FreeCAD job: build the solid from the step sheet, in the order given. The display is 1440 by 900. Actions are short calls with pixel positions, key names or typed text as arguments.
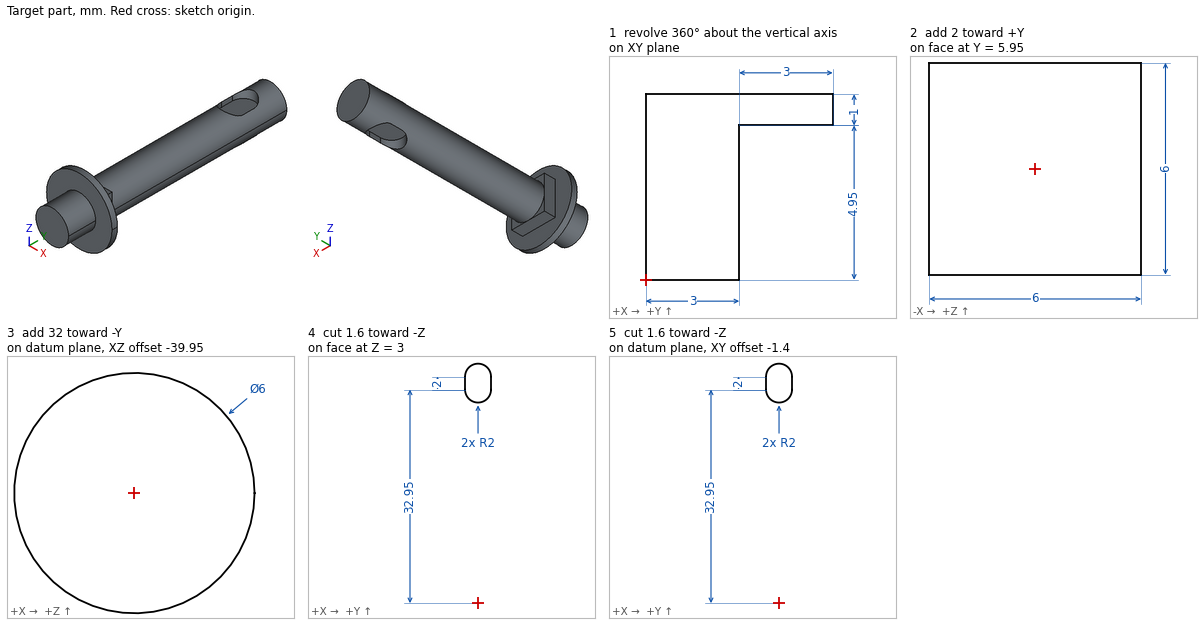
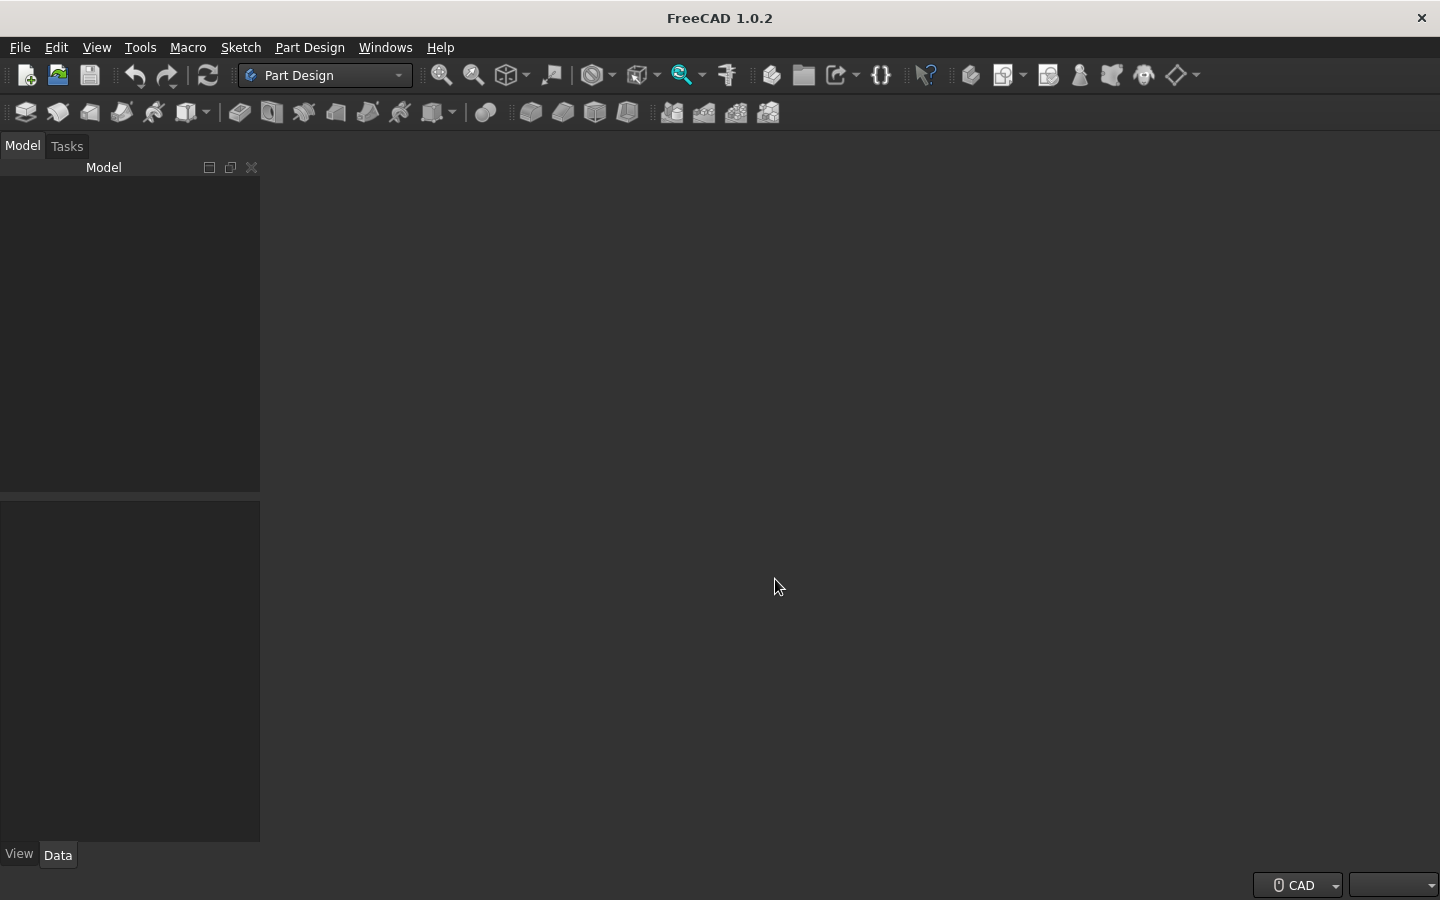
click(26, 76)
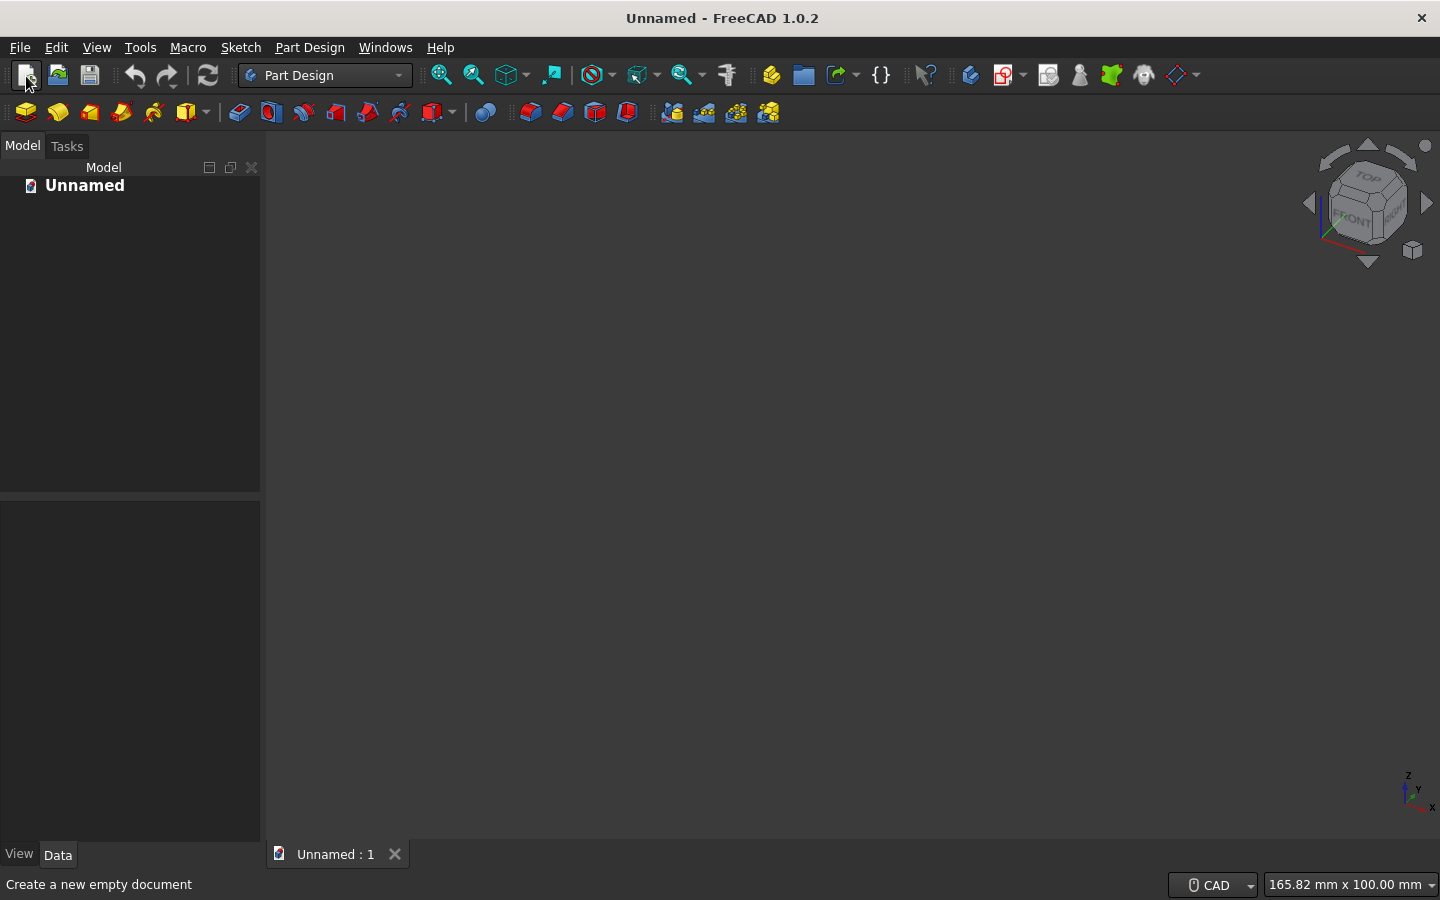
click(1004, 76)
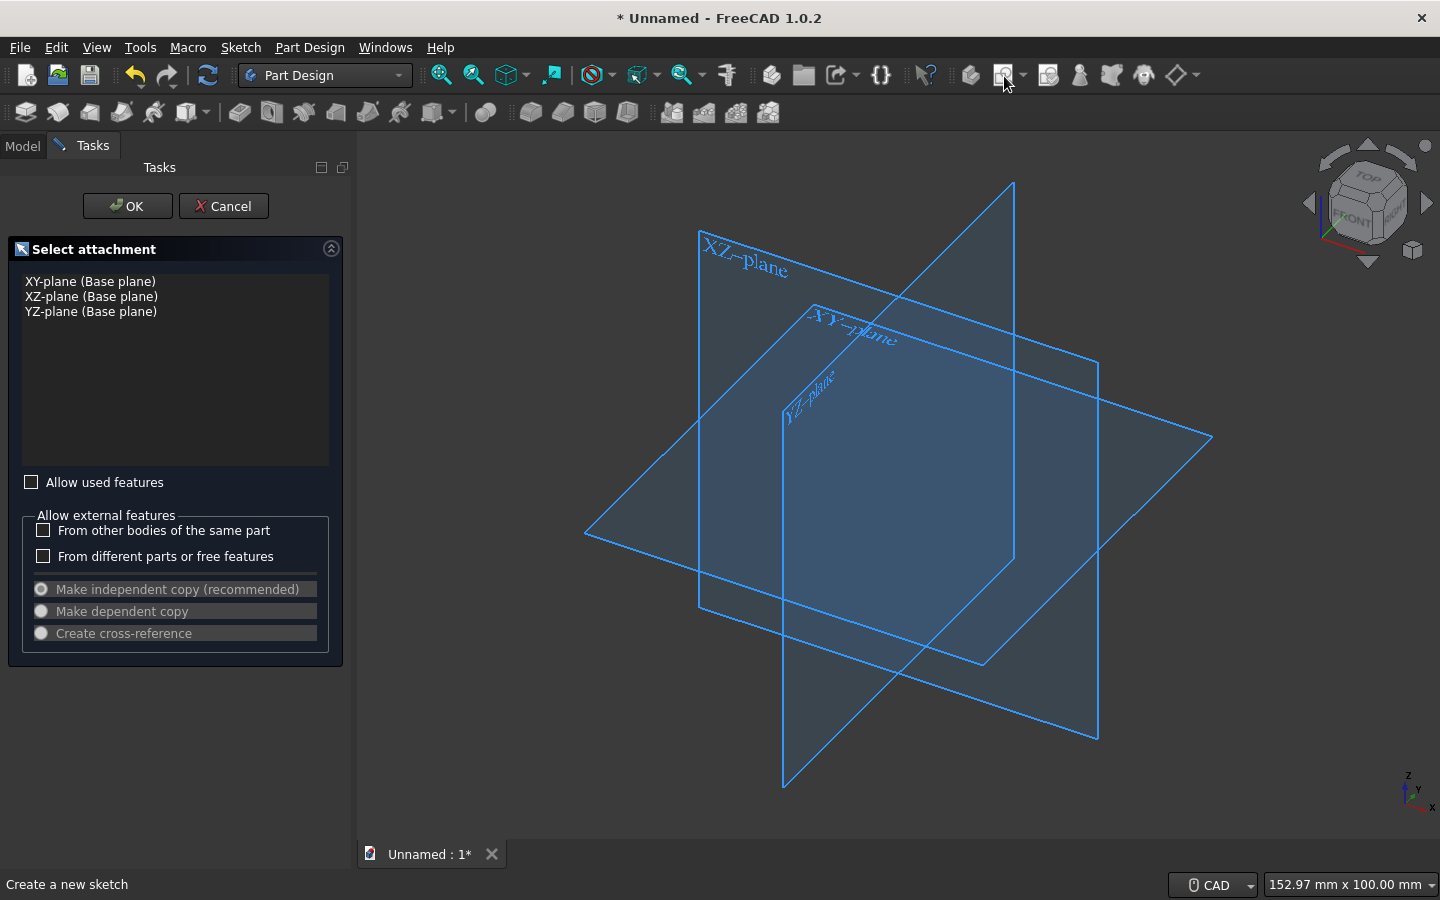
click(82, 282)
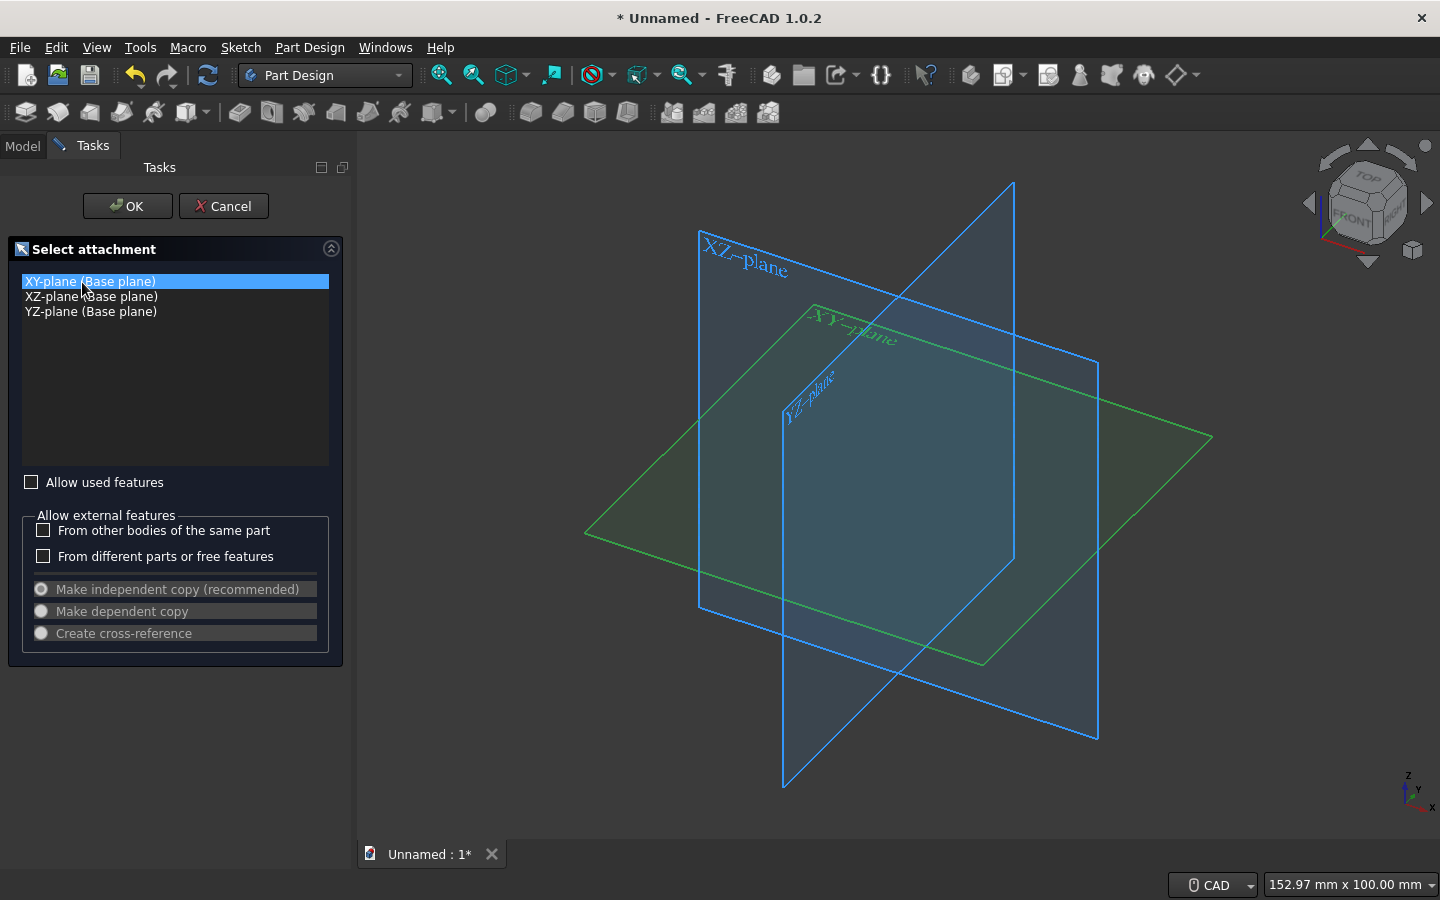
click(128, 206)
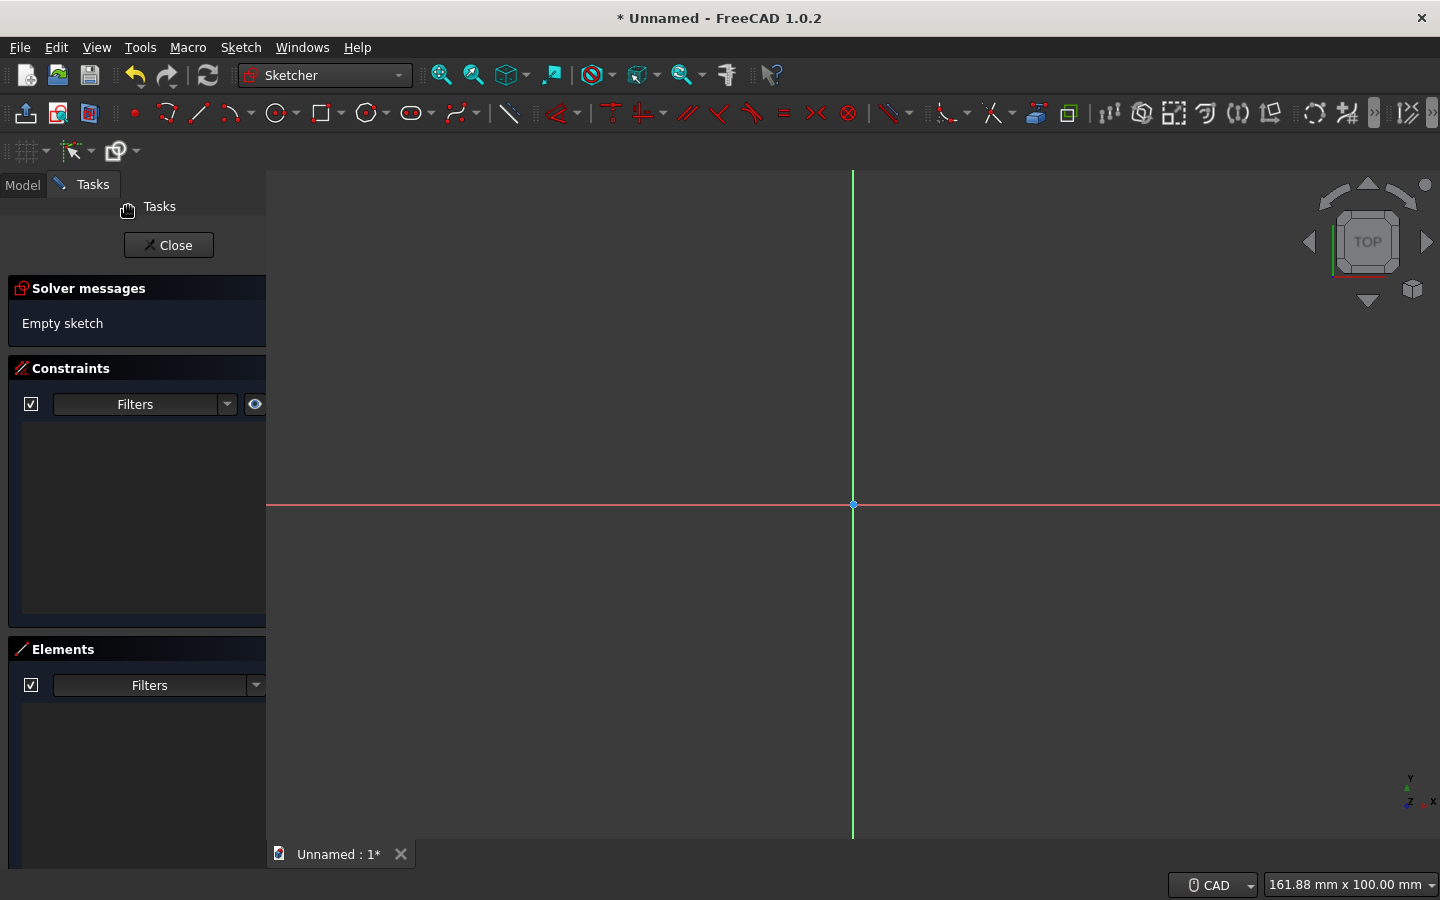
scroll(882, 483, up, 12)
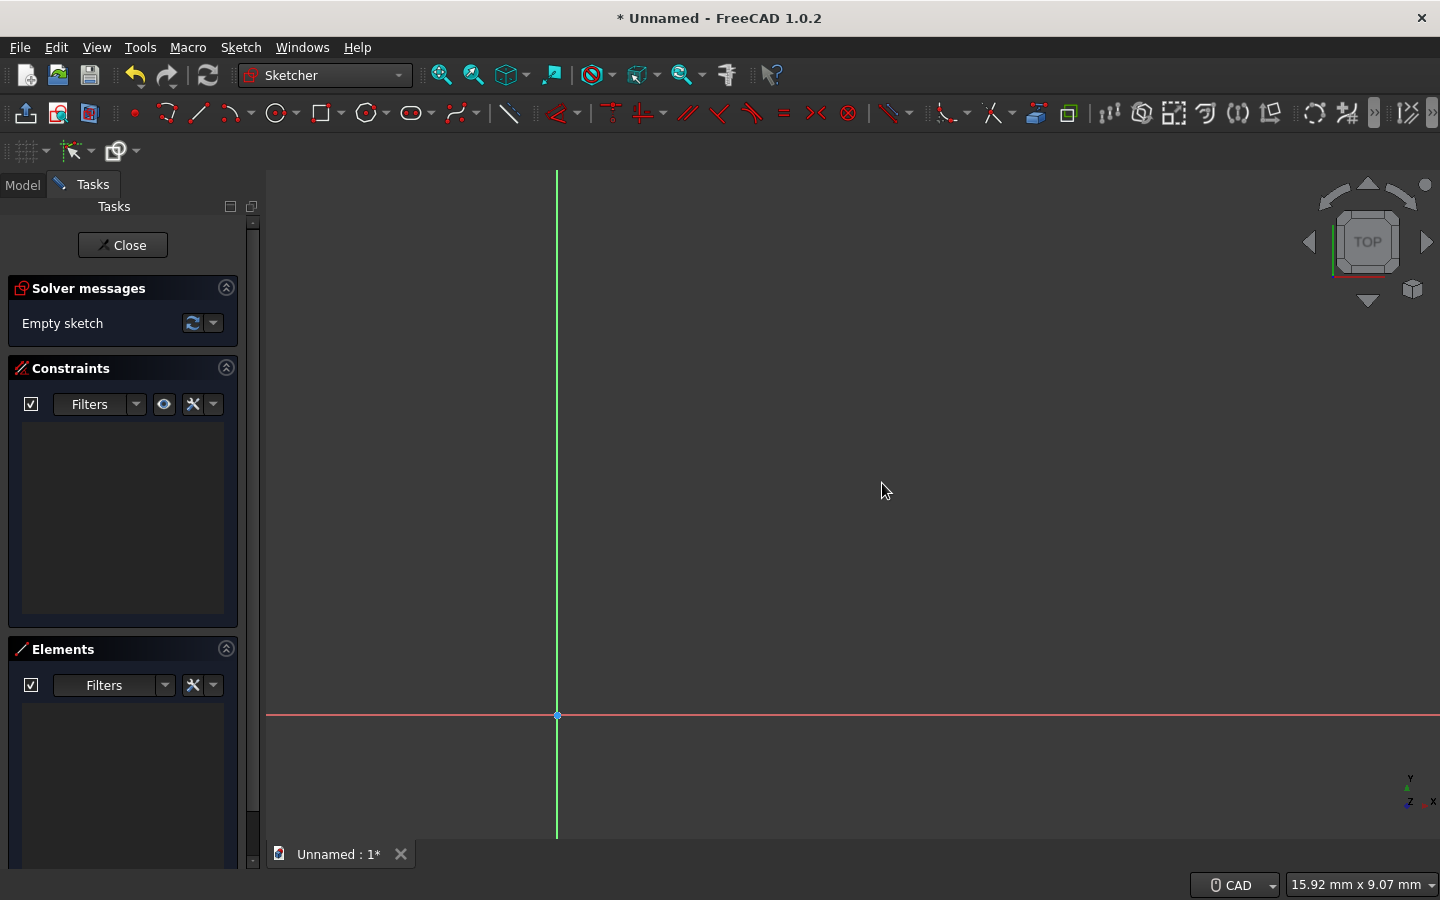
click(168, 114)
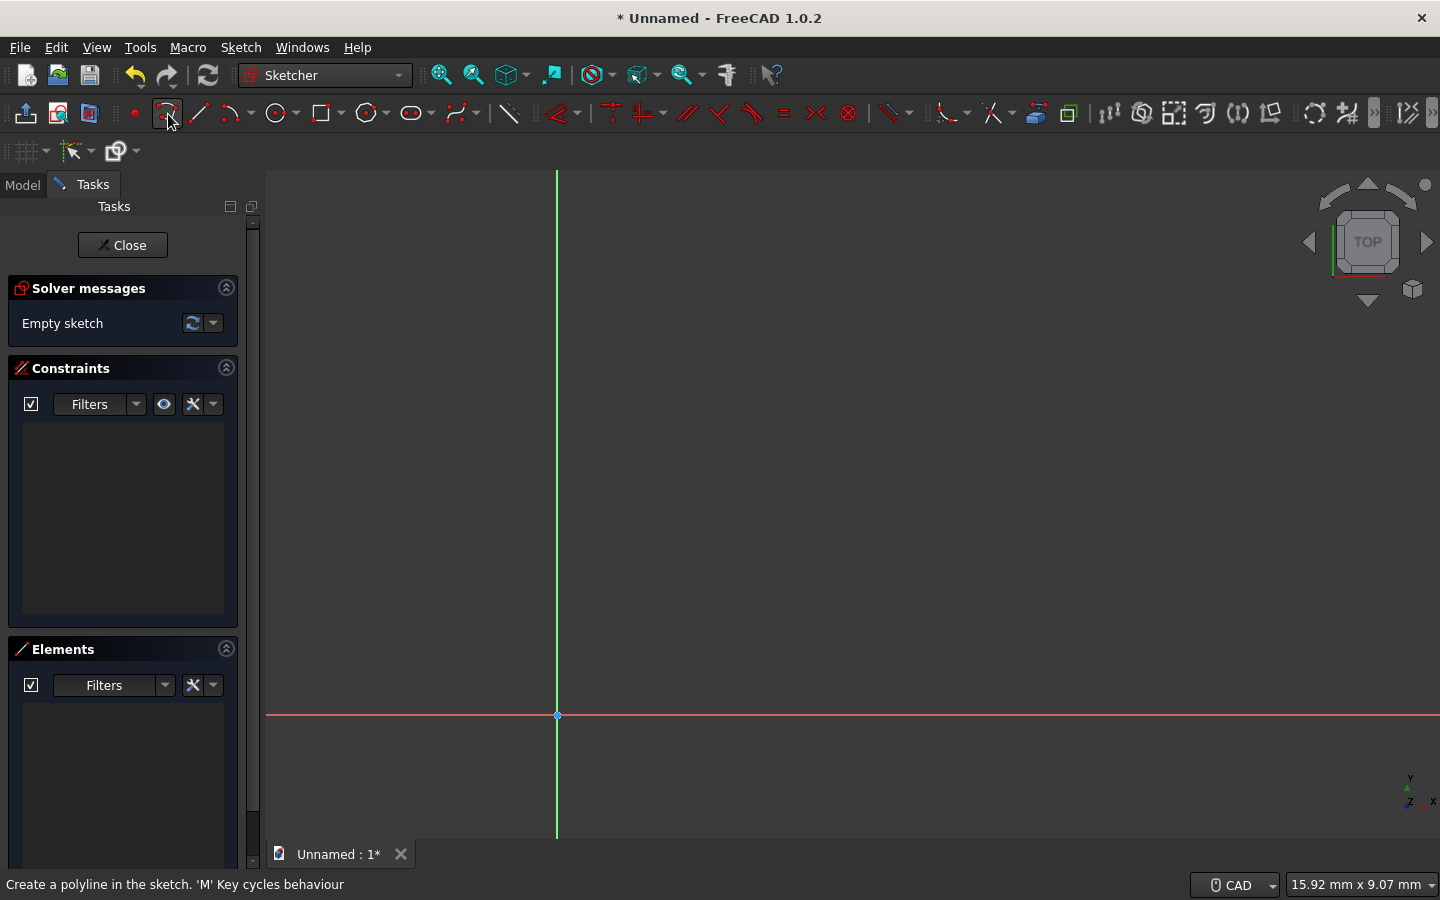
click(557, 715)
click(778, 706)
click(778, 350)
click(1000, 350)
click(1000, 277)
click(566, 277)
click(557, 715)
key(Escape)
key(Escape)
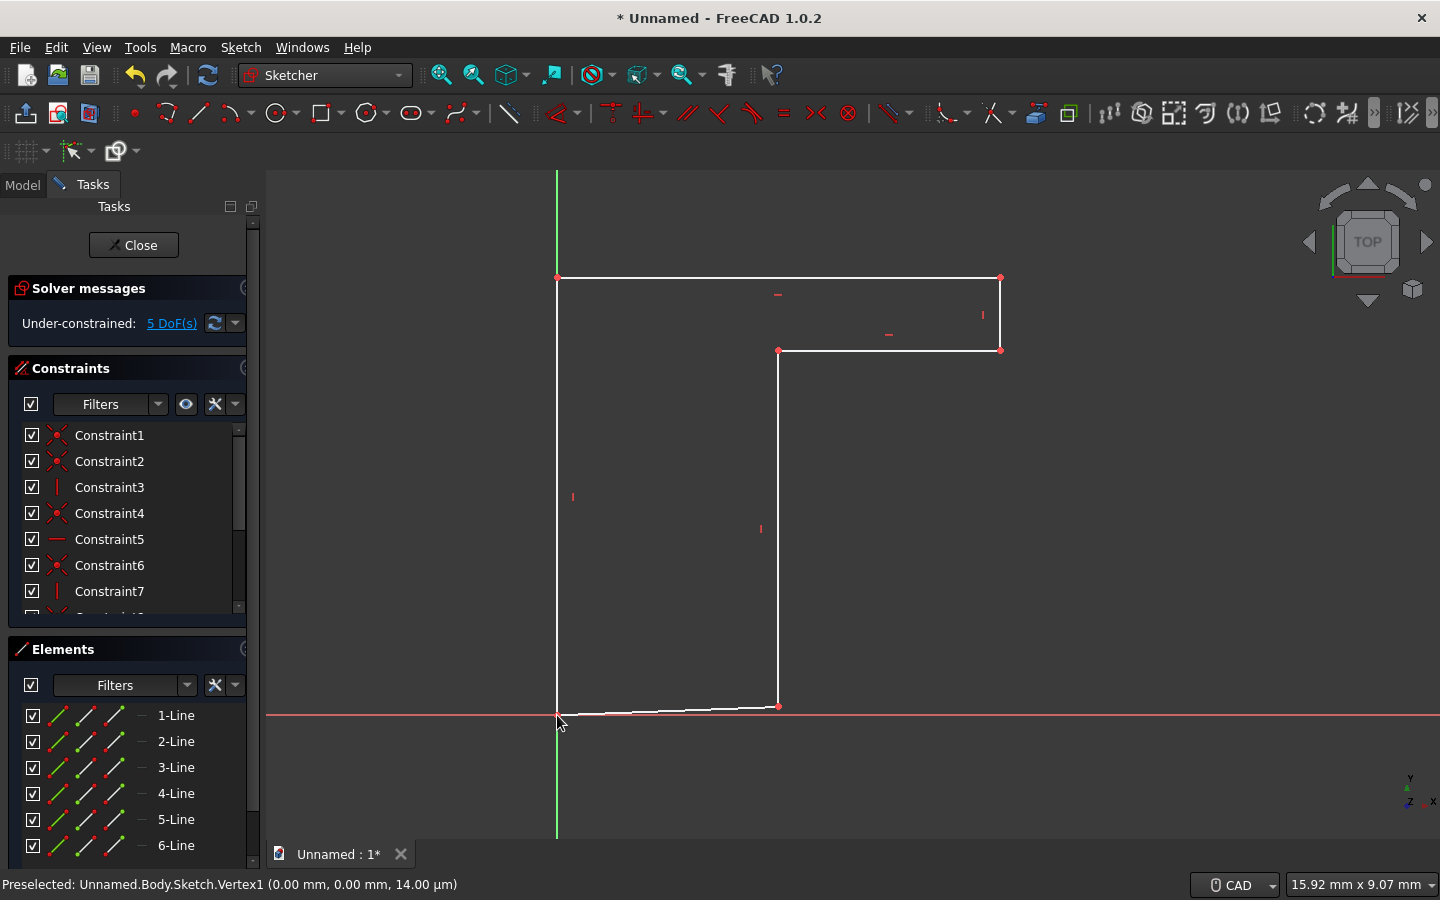
click(623, 713)